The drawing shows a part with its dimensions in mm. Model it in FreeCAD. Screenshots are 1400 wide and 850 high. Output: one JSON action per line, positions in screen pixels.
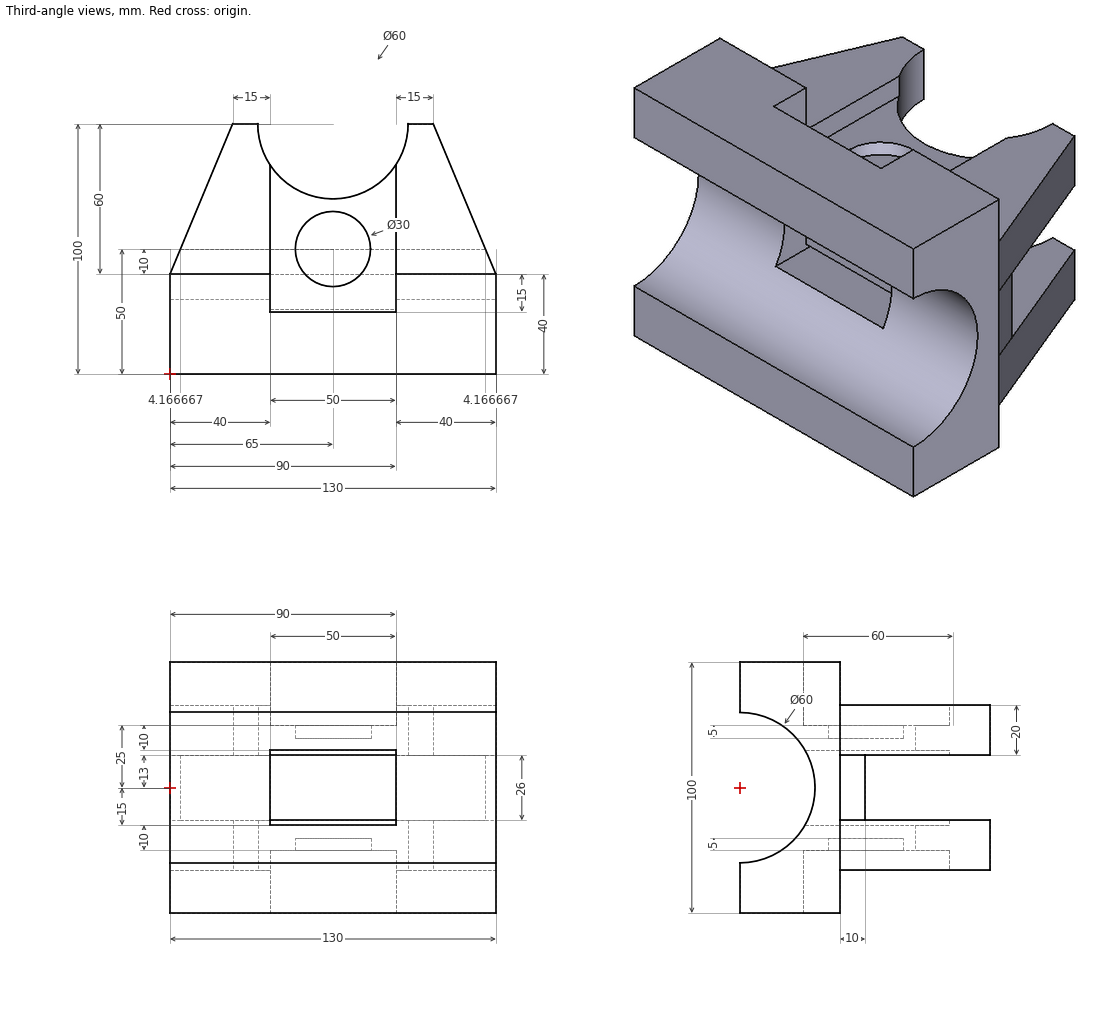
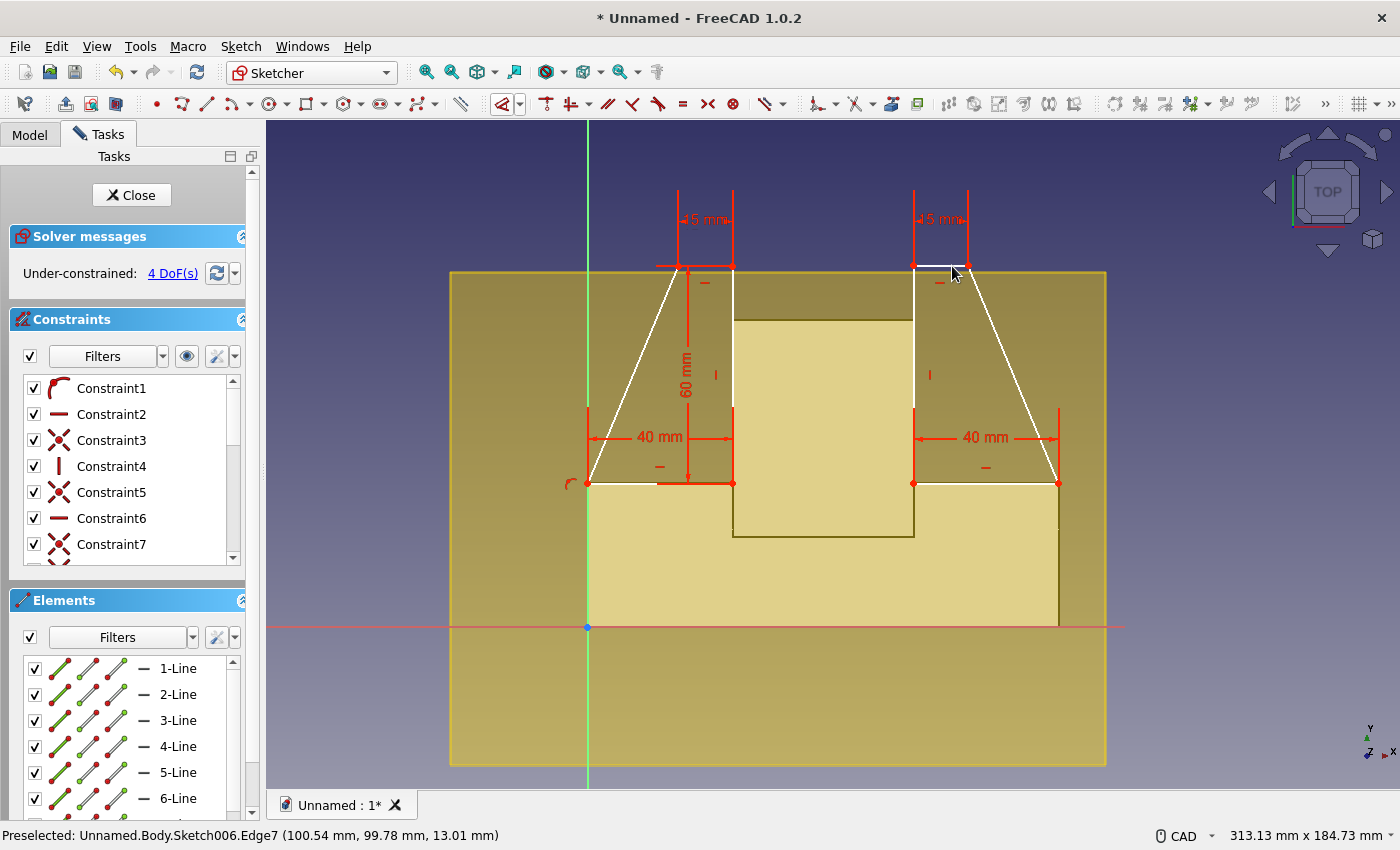
{"action": "left_click", "coordinate": [914, 331]}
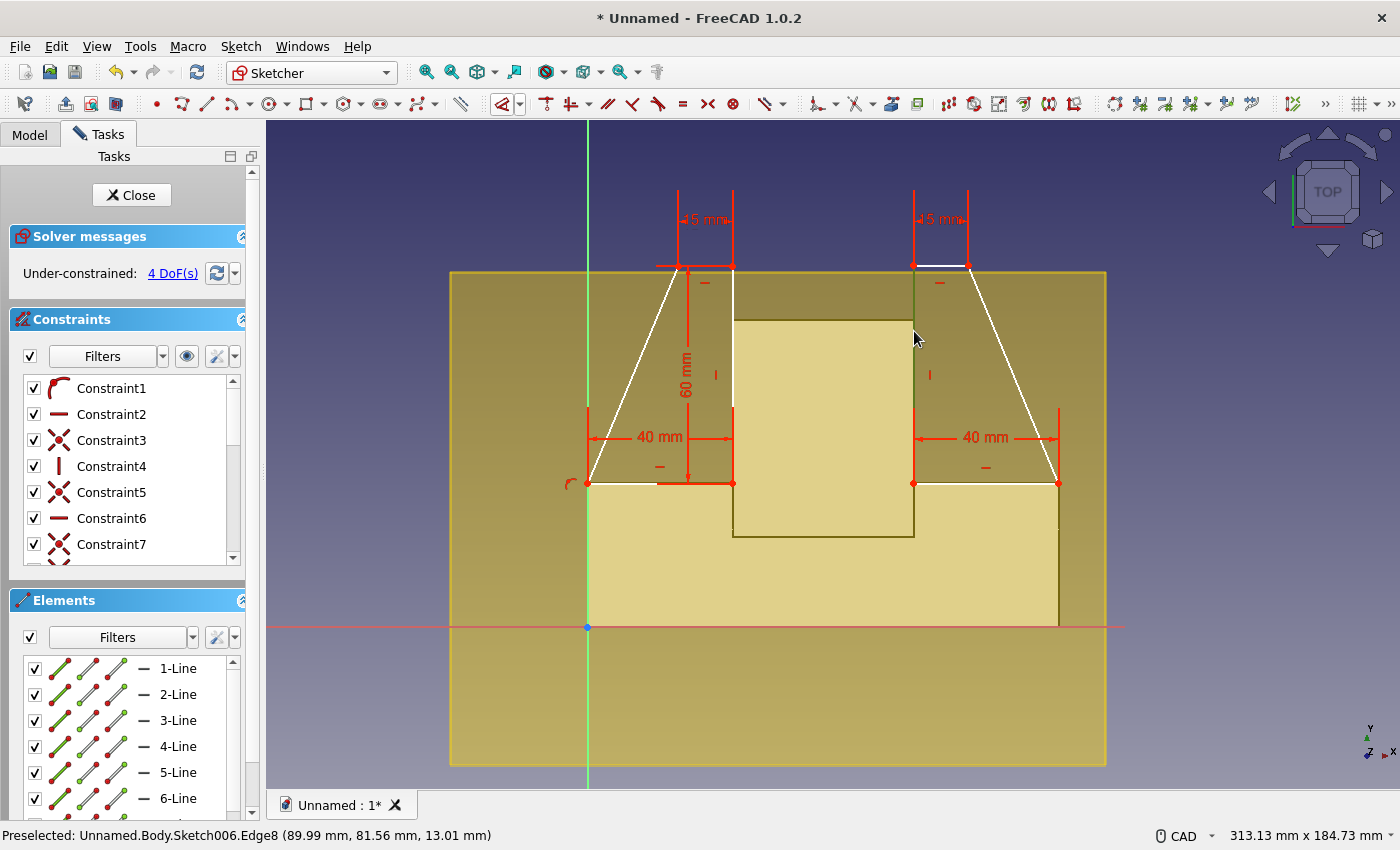
{"action": "left_click", "coordinate": [520, 104]}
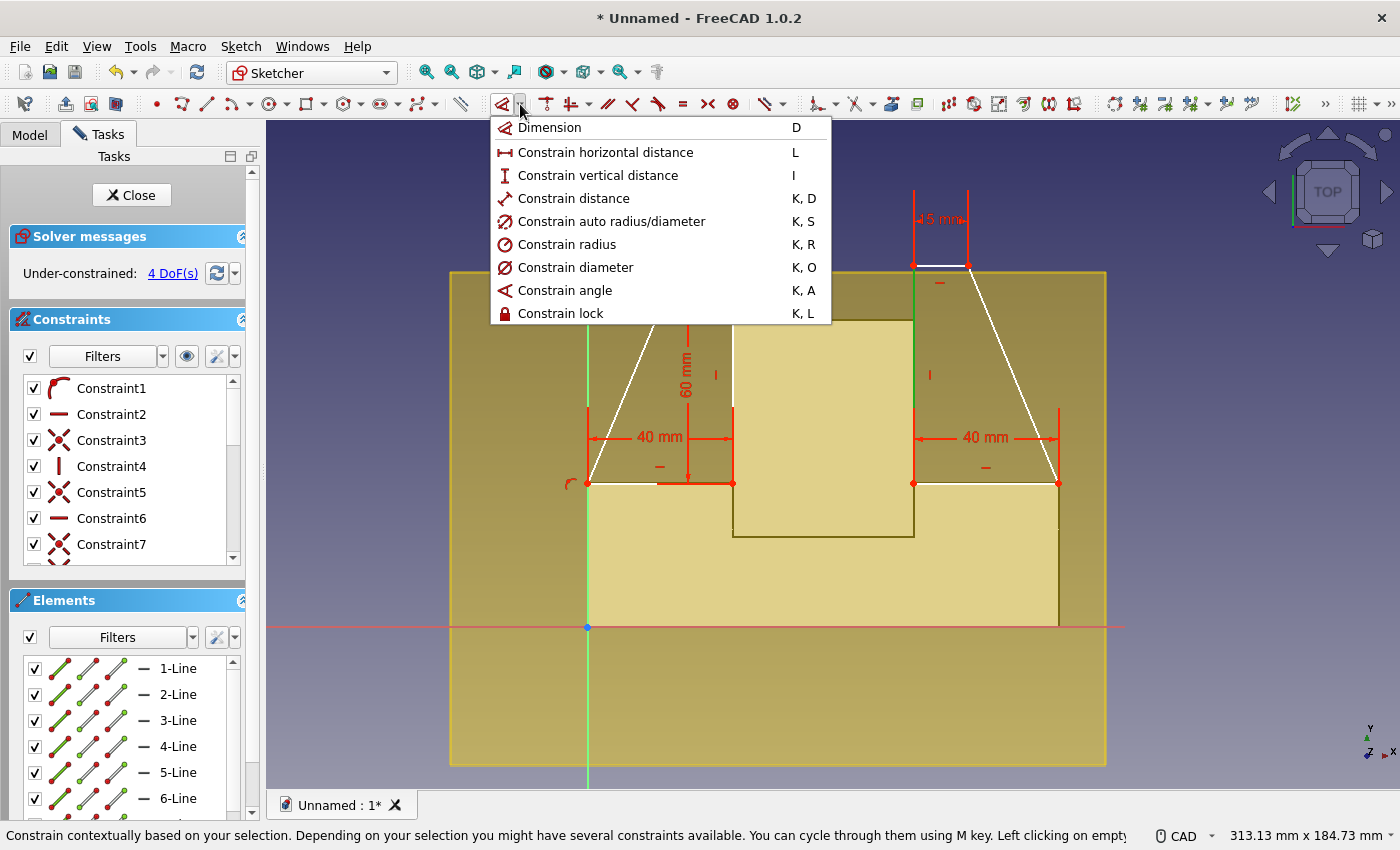
{"action": "left_click", "coordinate": [661, 176]}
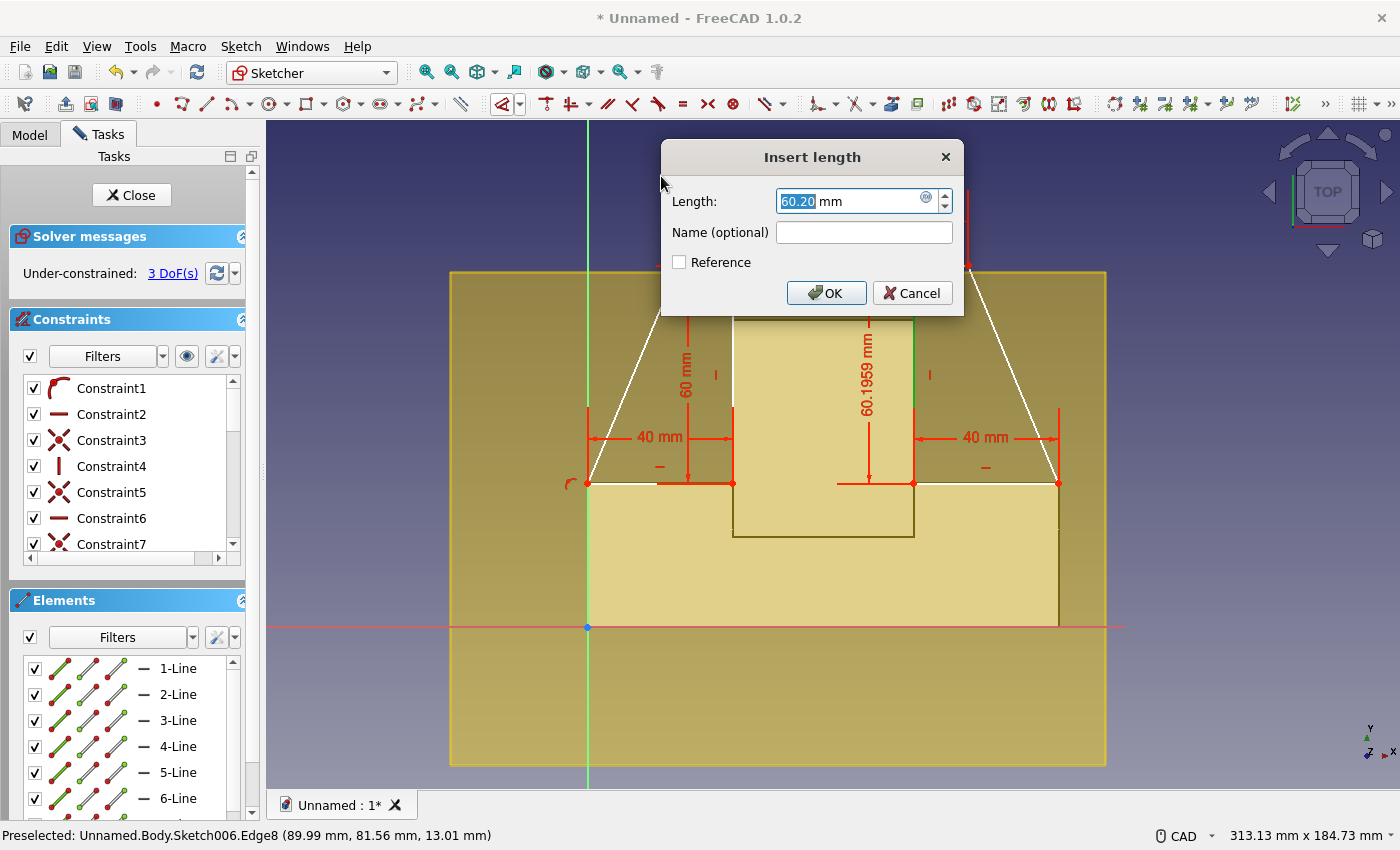
{"action": "type", "text": "60"}
{"action": "key", "text": "Return"}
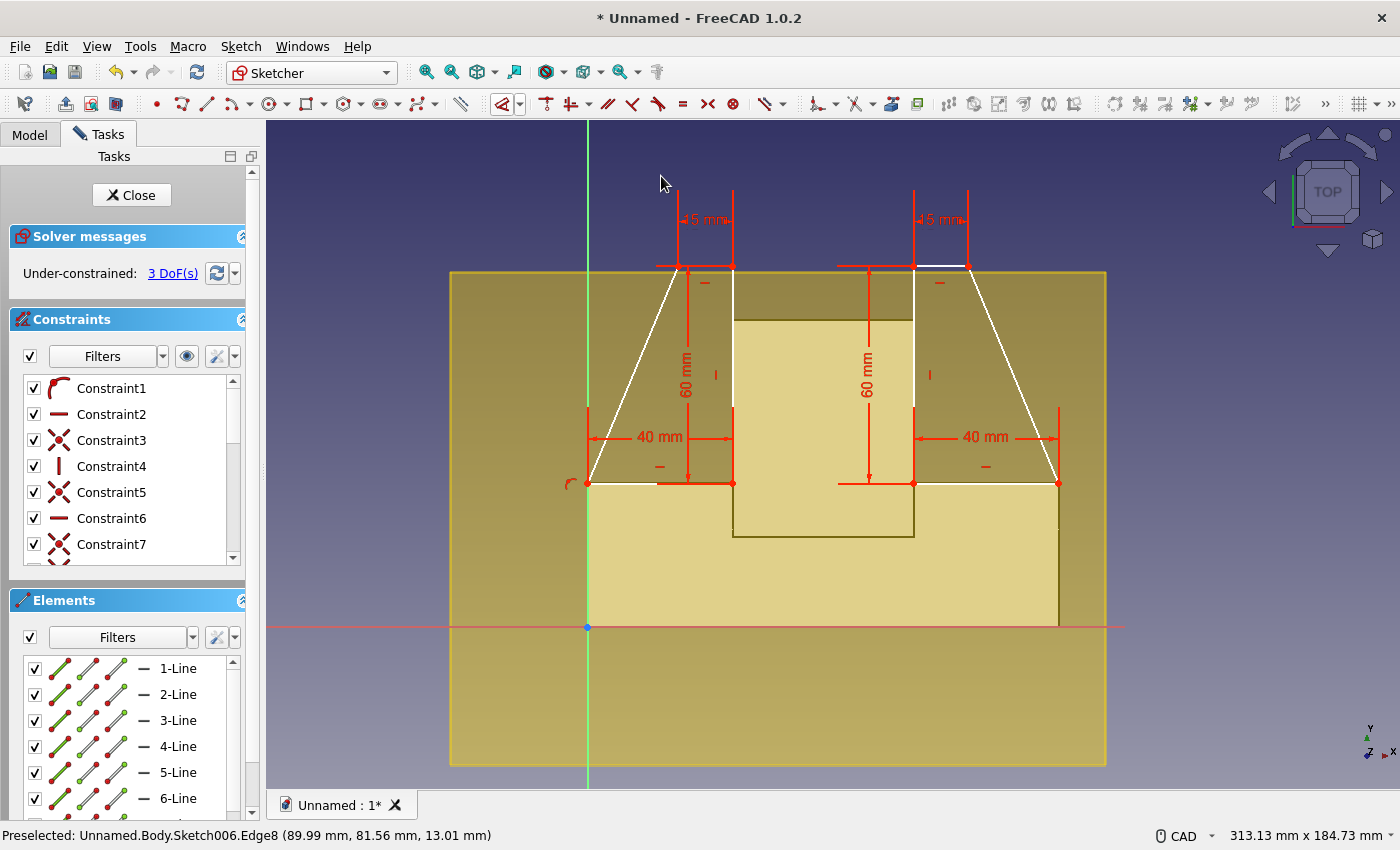
{"action": "left_click", "coordinate": [588, 484]}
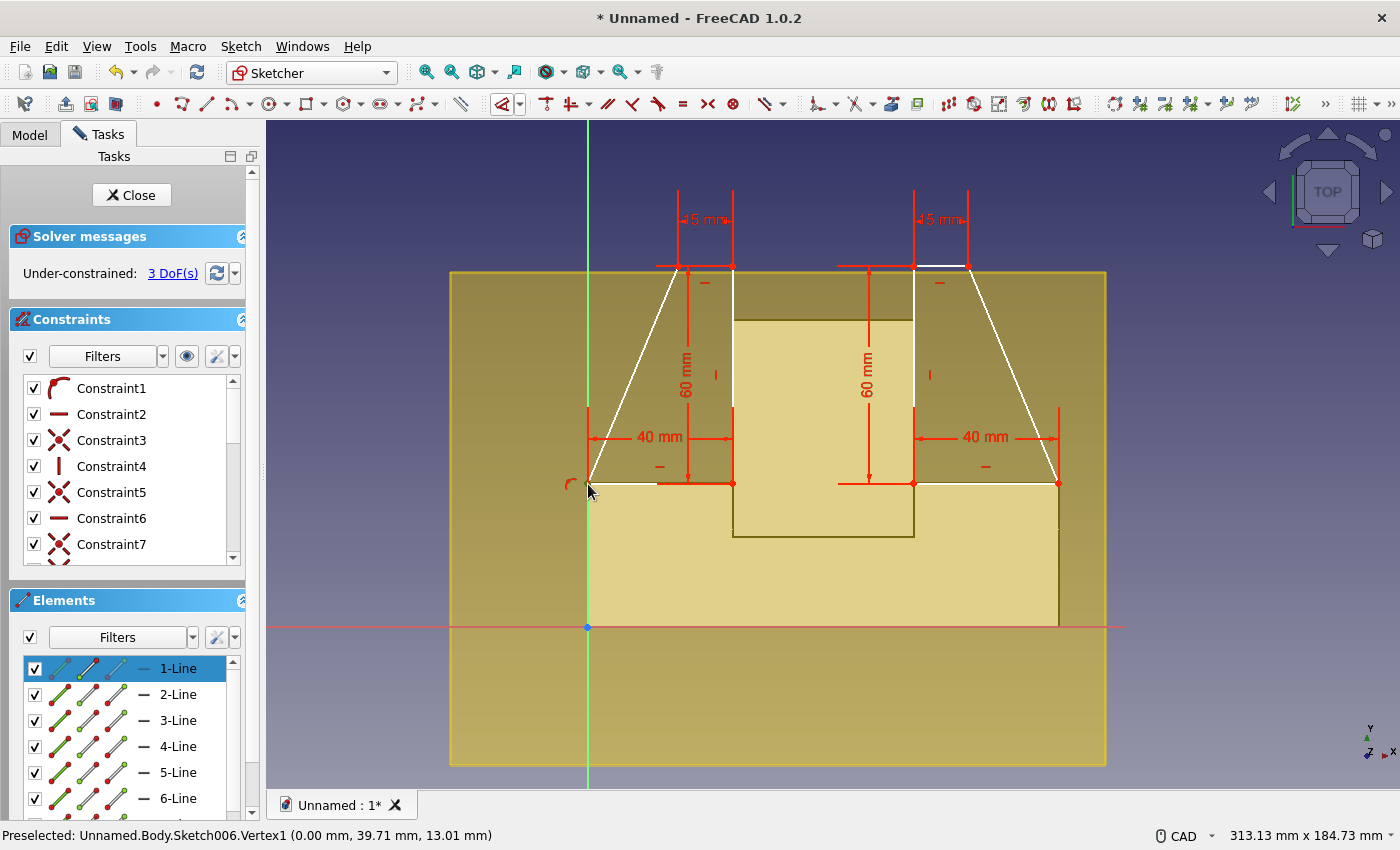
{"action": "key", "text": "i"}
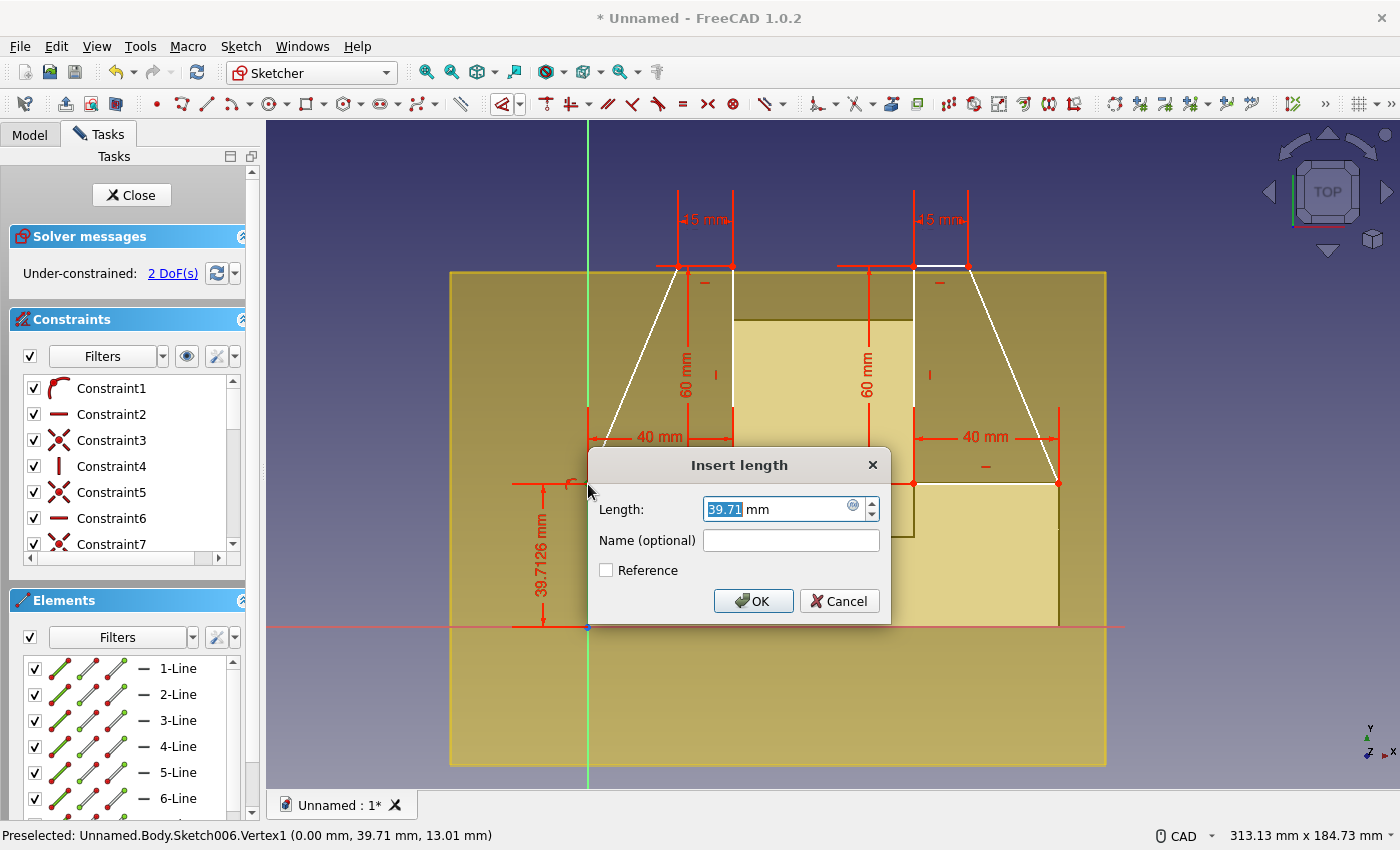
{"action": "type", "text": "40"}
{"action": "key", "text": "Return"}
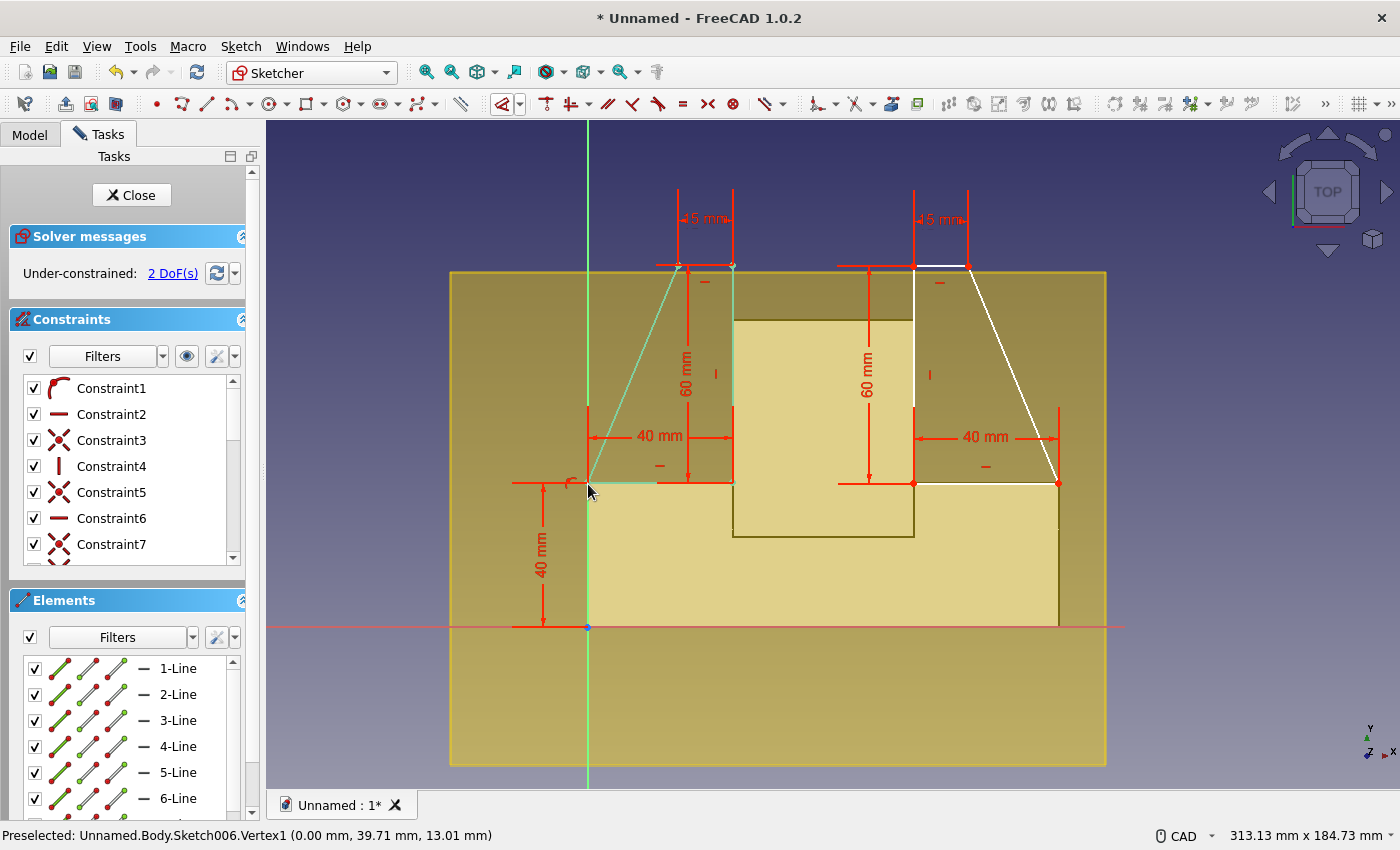
{"action": "left_click", "coordinate": [914, 484]}